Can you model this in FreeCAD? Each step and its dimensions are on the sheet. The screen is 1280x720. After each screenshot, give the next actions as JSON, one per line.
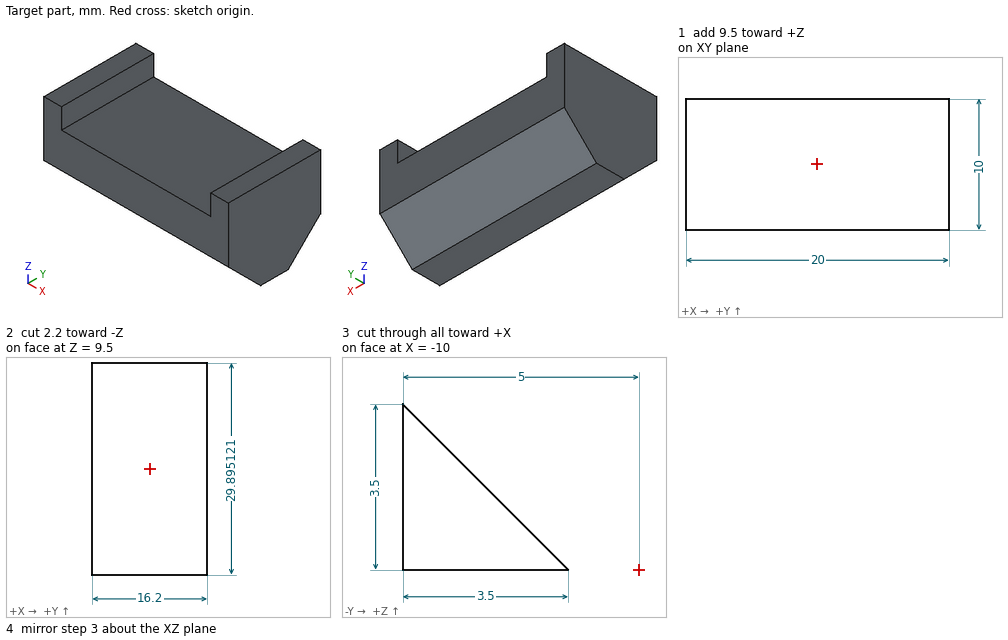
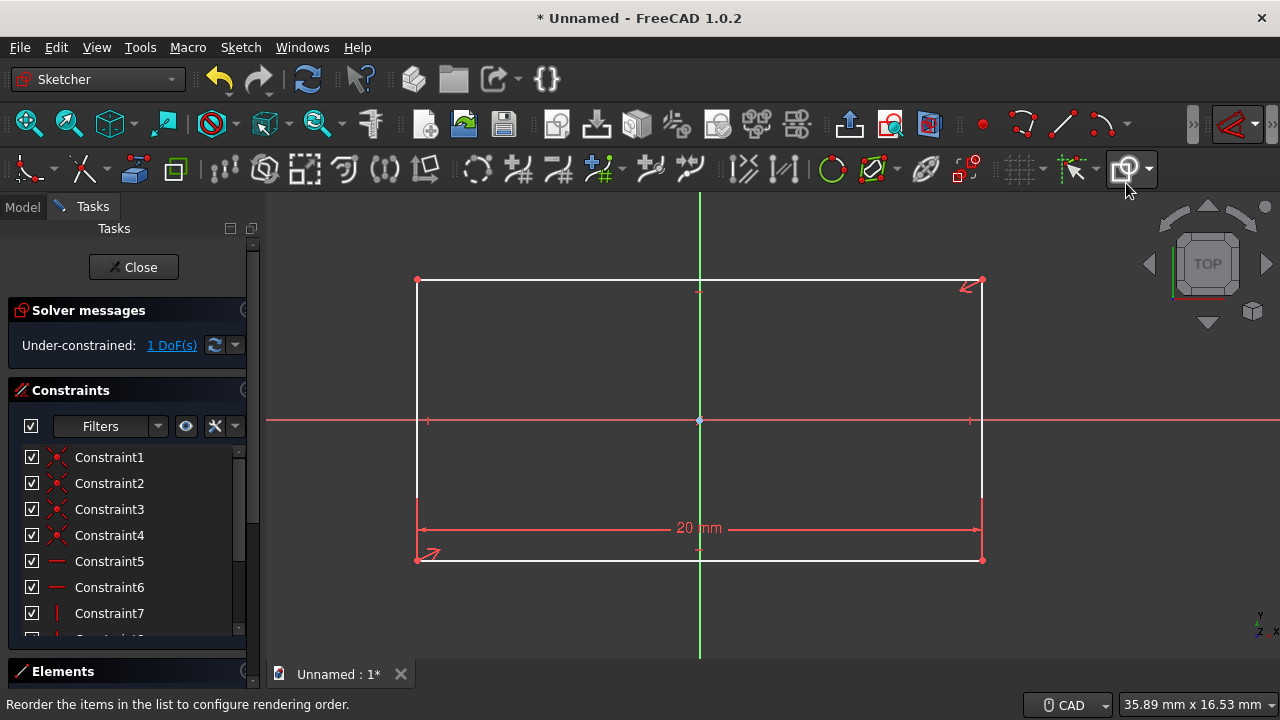
{"action": "left_click", "coordinate": [982, 477]}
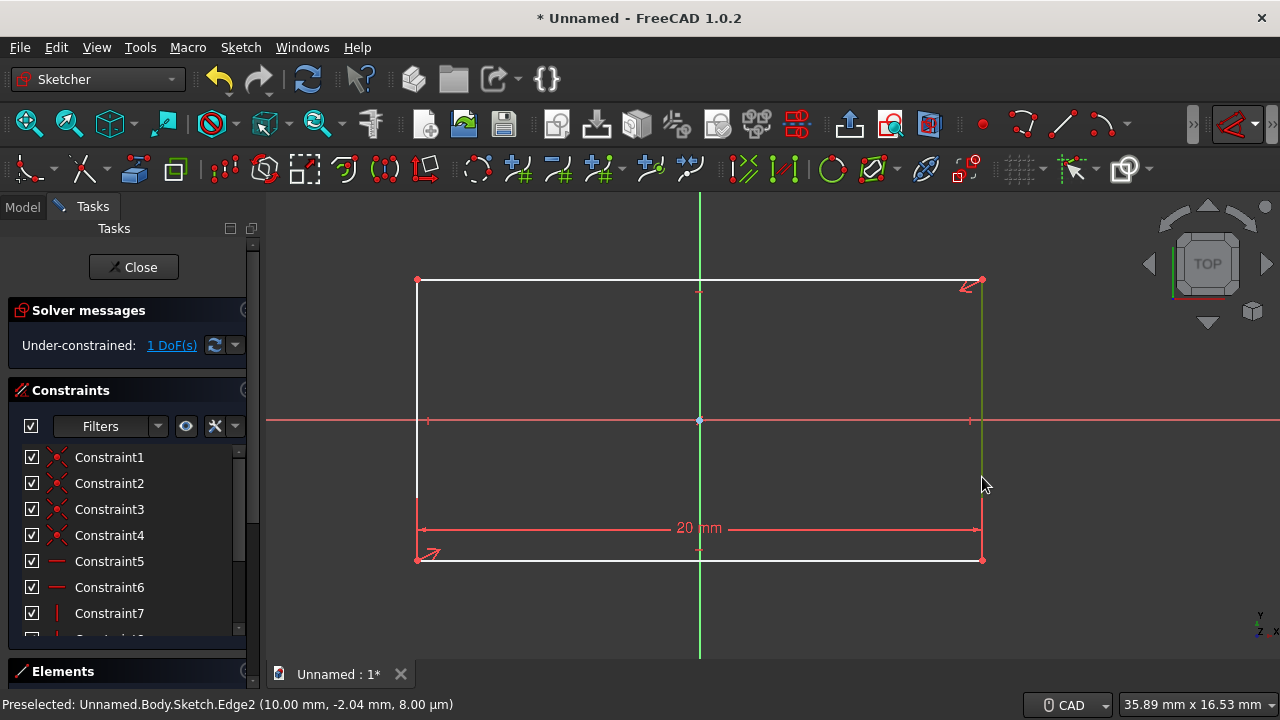
{"action": "left_click", "coordinate": [1258, 124]}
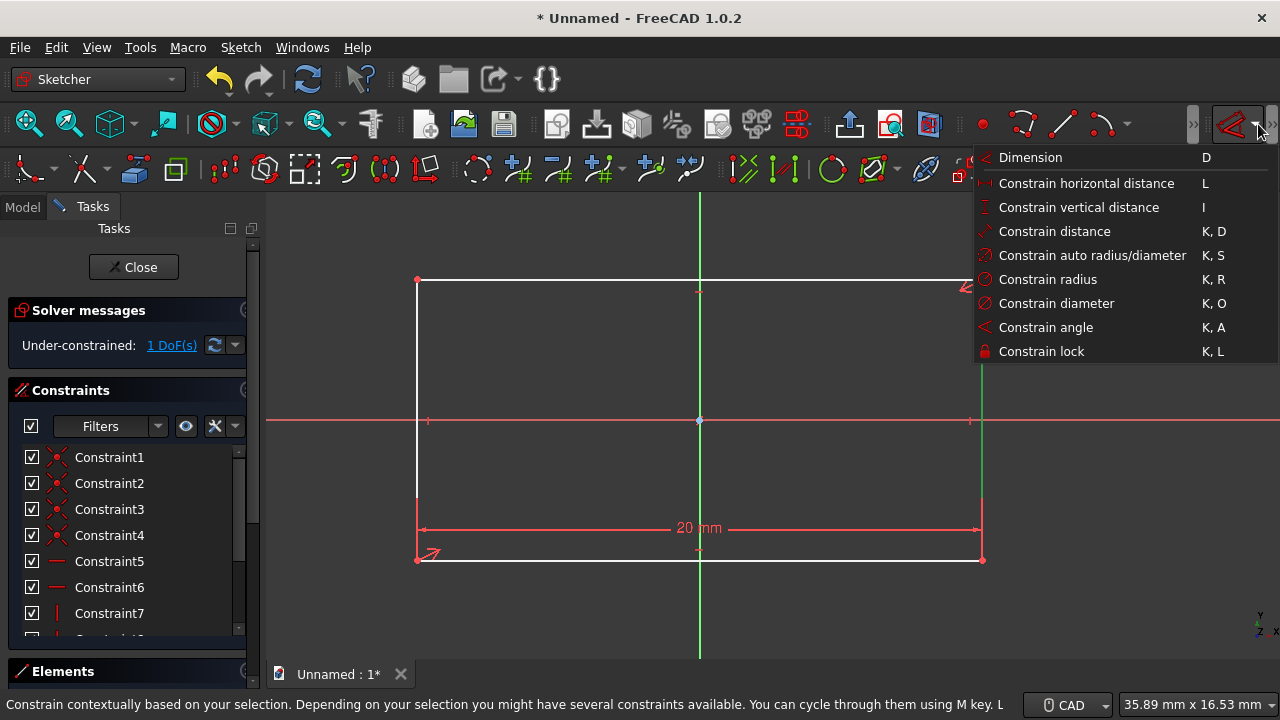
{"action": "left_click", "coordinate": [1126, 207]}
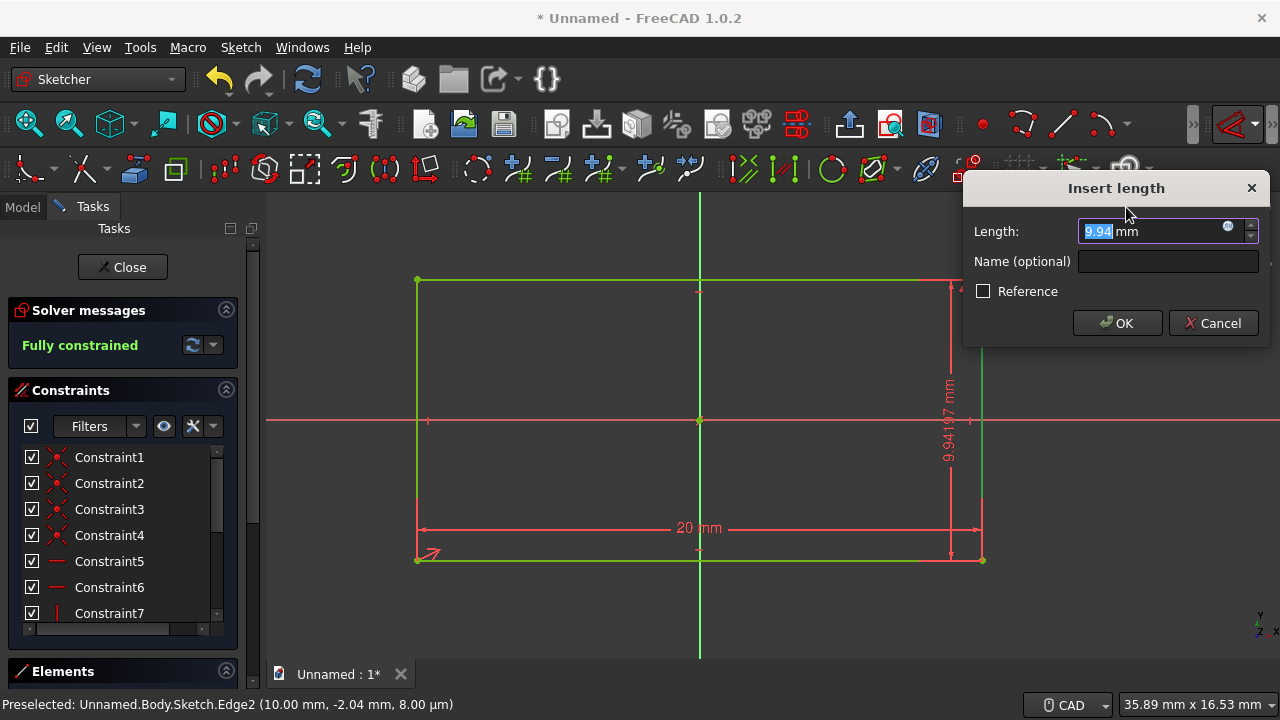
{"action": "type", "text": "10"}
{"action": "key", "text": "Return"}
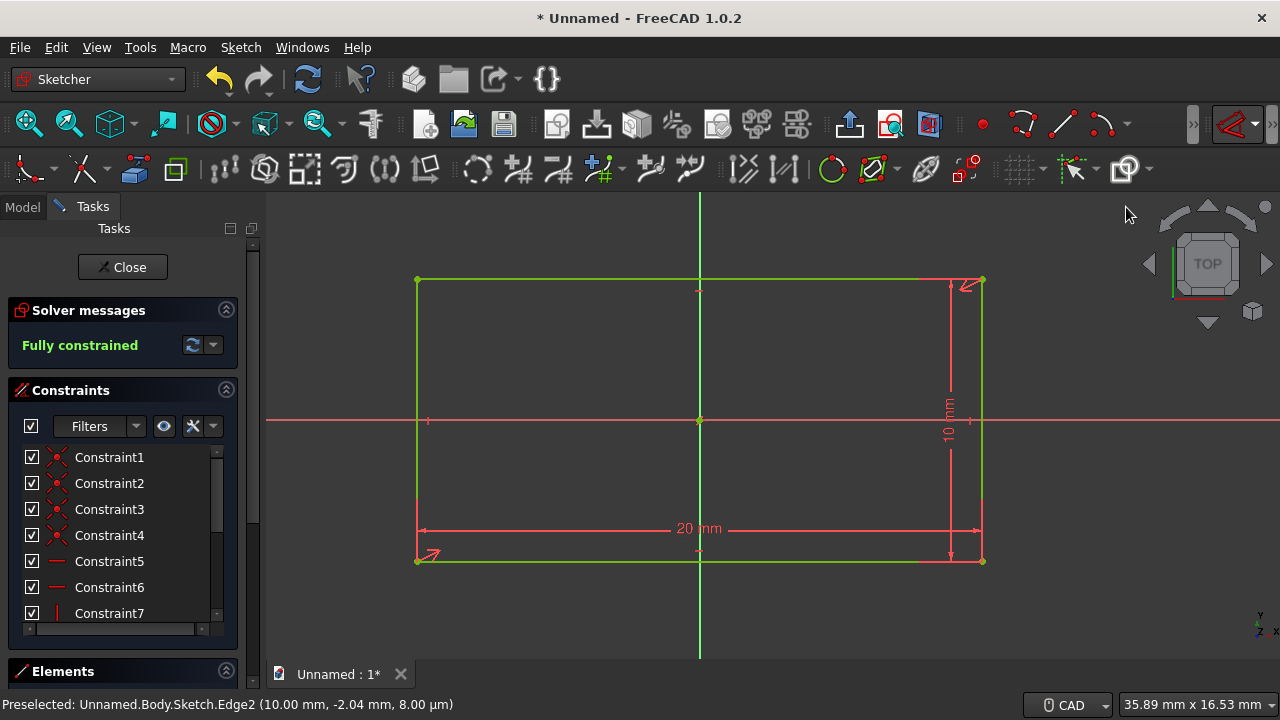
{"action": "left_click", "coordinate": [123, 267]}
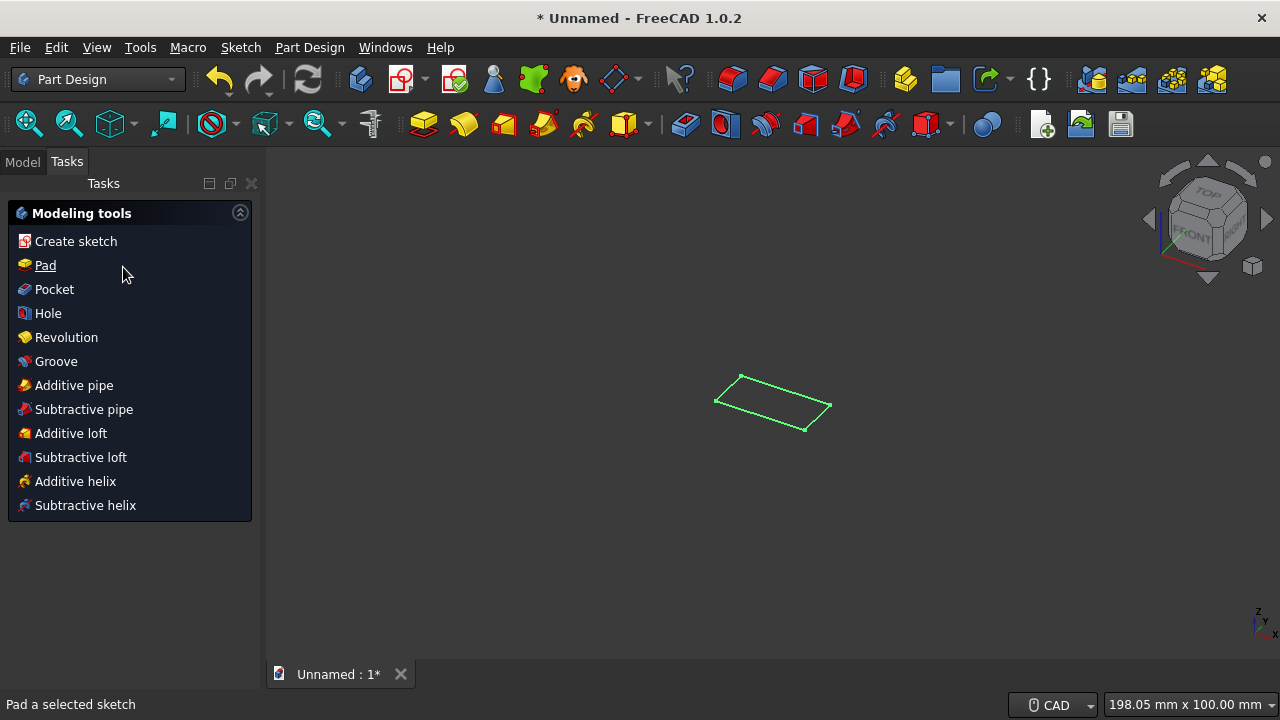
{"action": "left_click", "coordinate": [424, 124]}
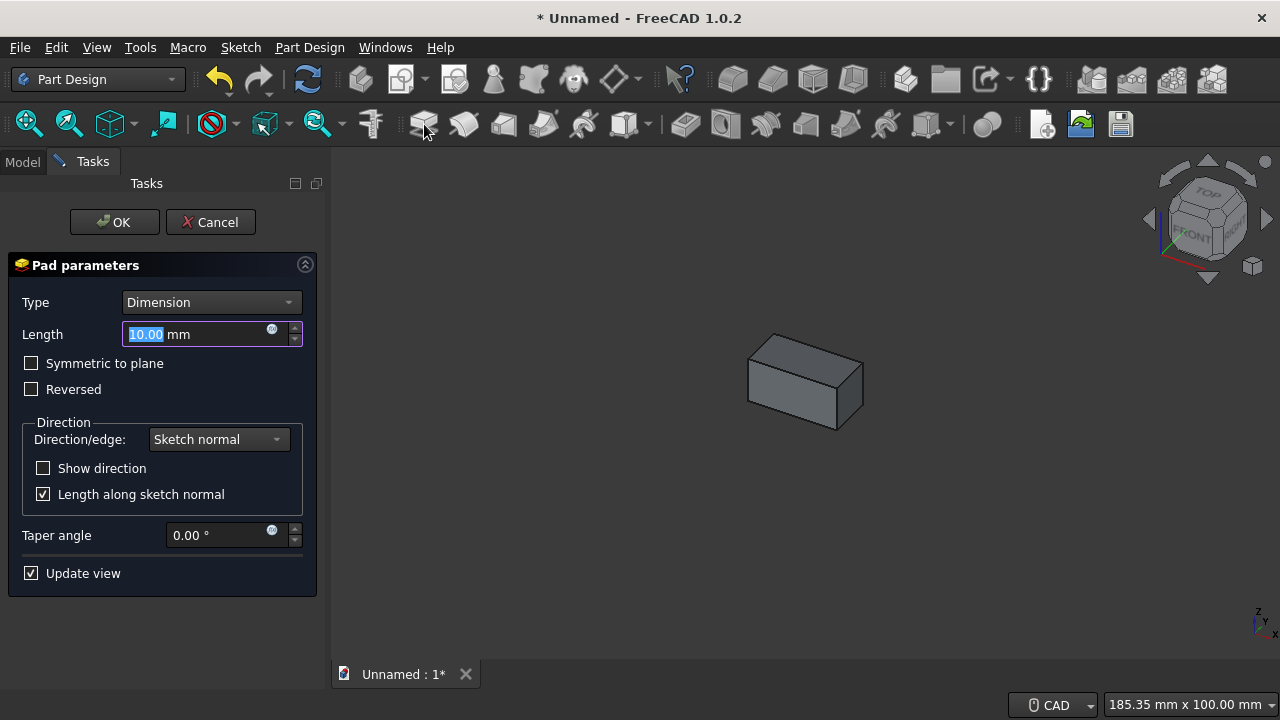
{"action": "type", "text": "9.5"}
{"action": "key", "text": "Tab"}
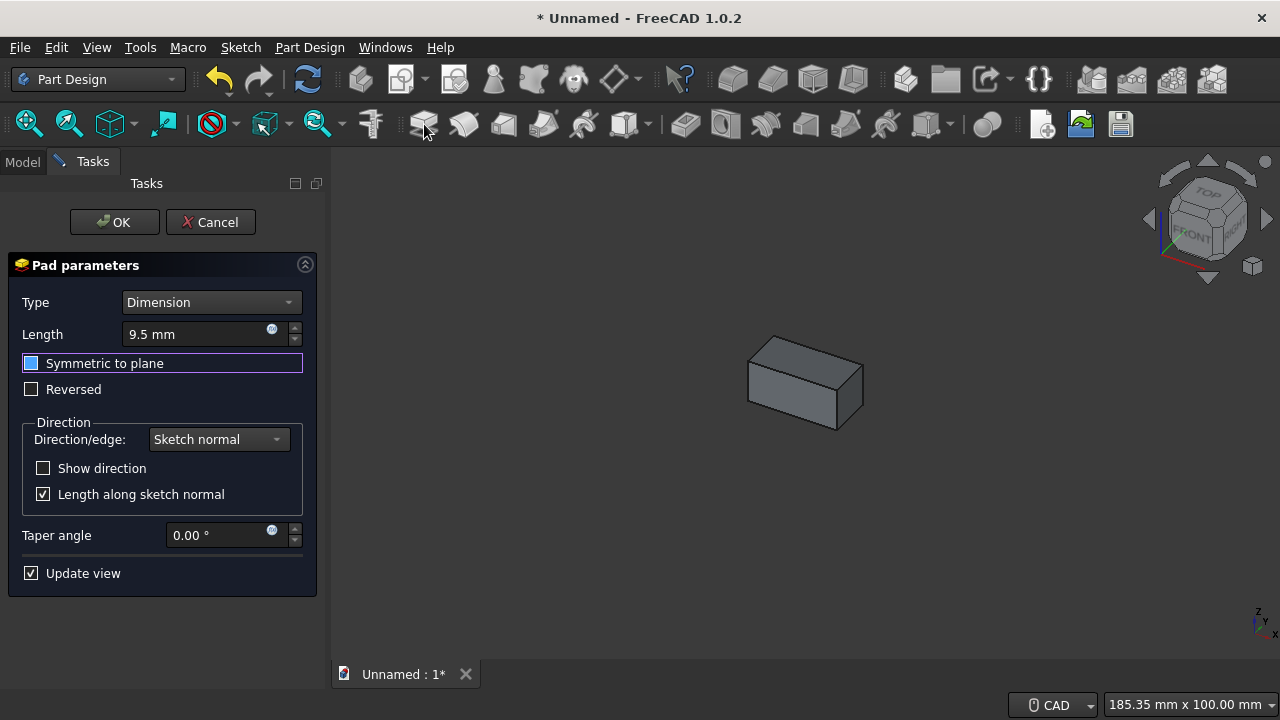
{"action": "left_click", "coordinate": [115, 222]}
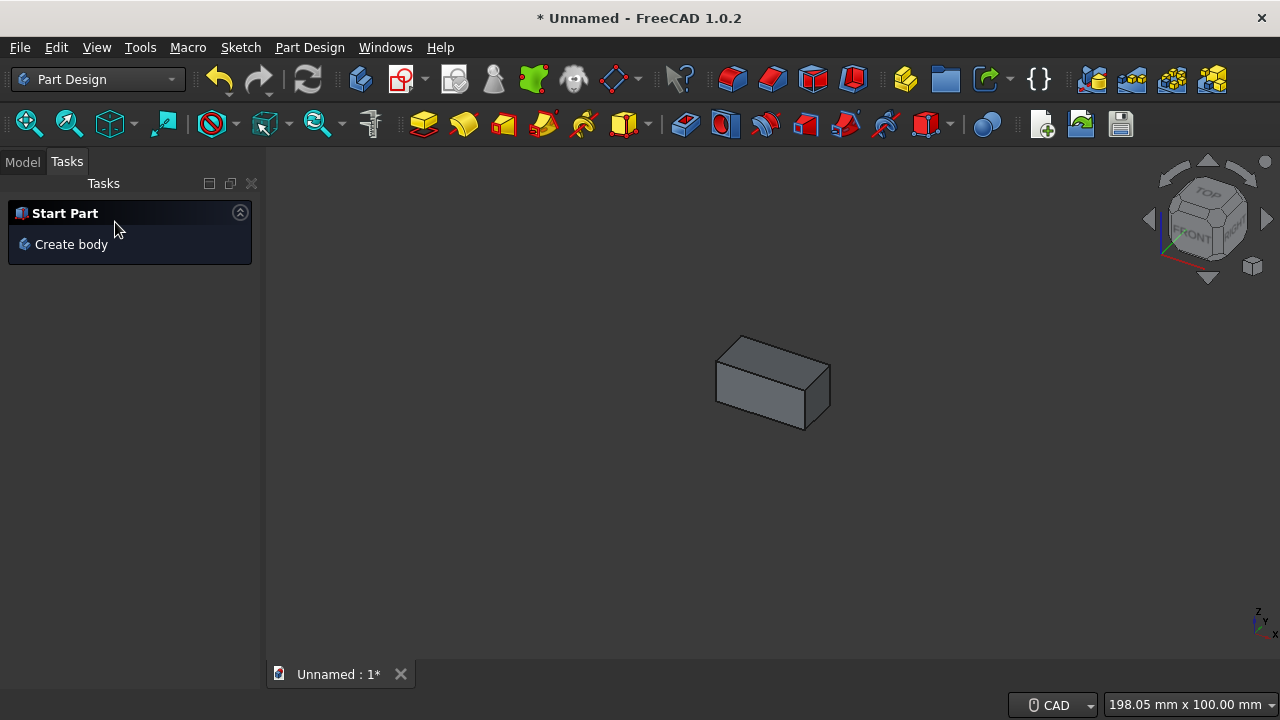
{"action": "key", "text": "v f"}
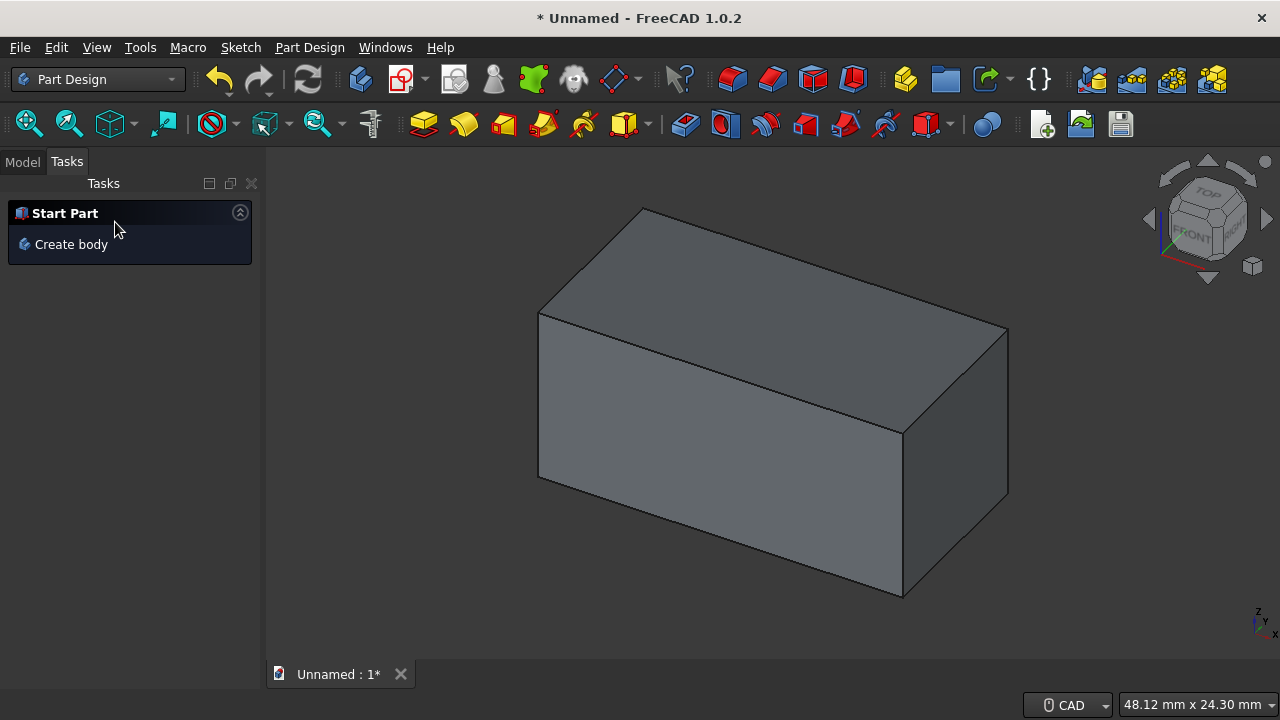
{"action": "left_click", "coordinate": [825, 337]}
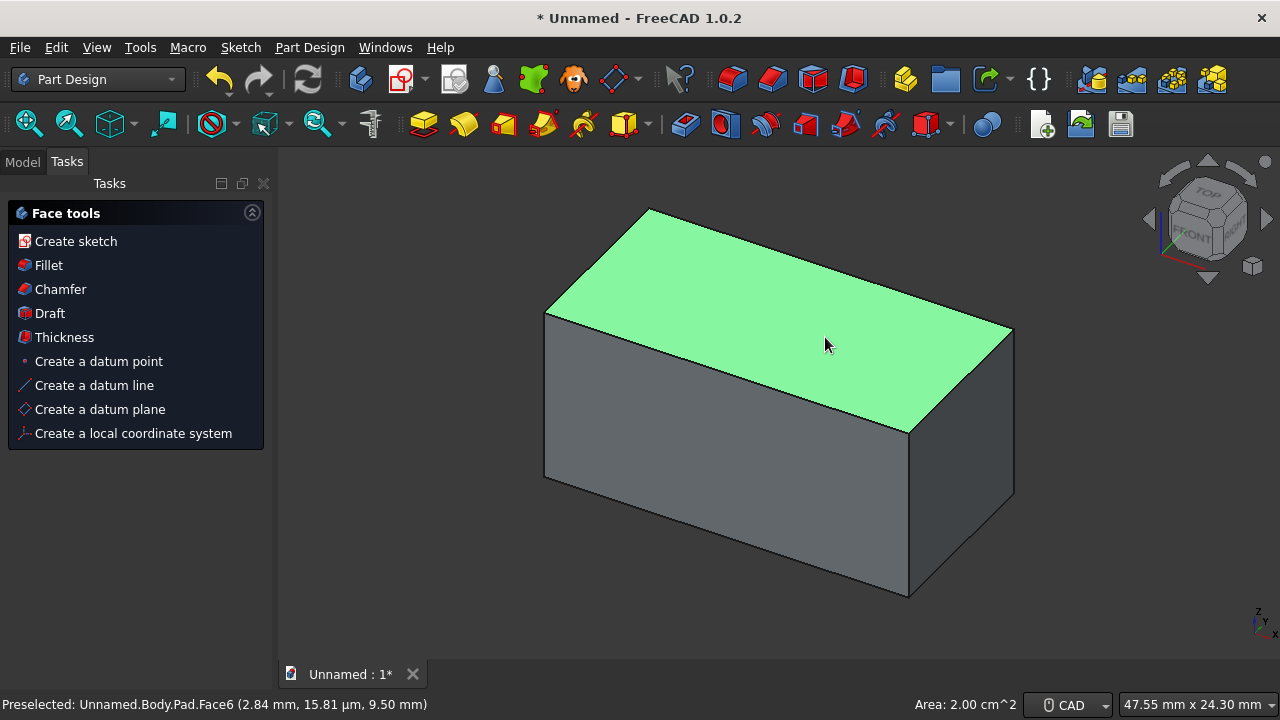
{"action": "left_click", "coordinate": [402, 80]}